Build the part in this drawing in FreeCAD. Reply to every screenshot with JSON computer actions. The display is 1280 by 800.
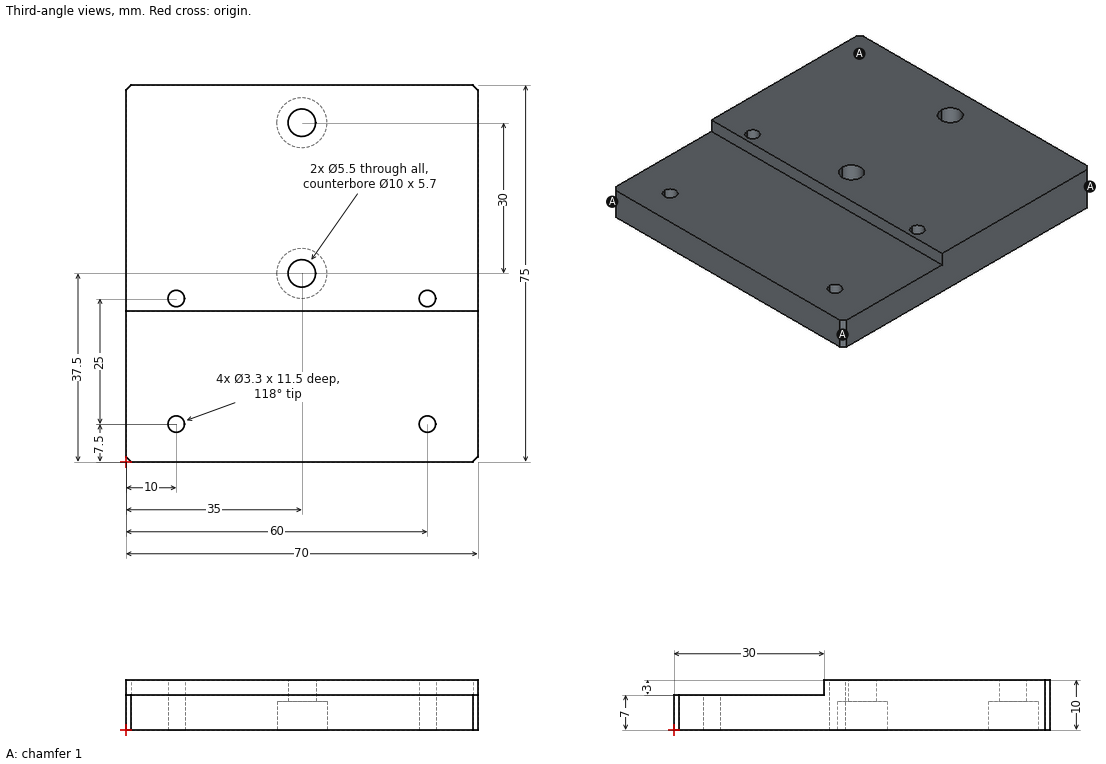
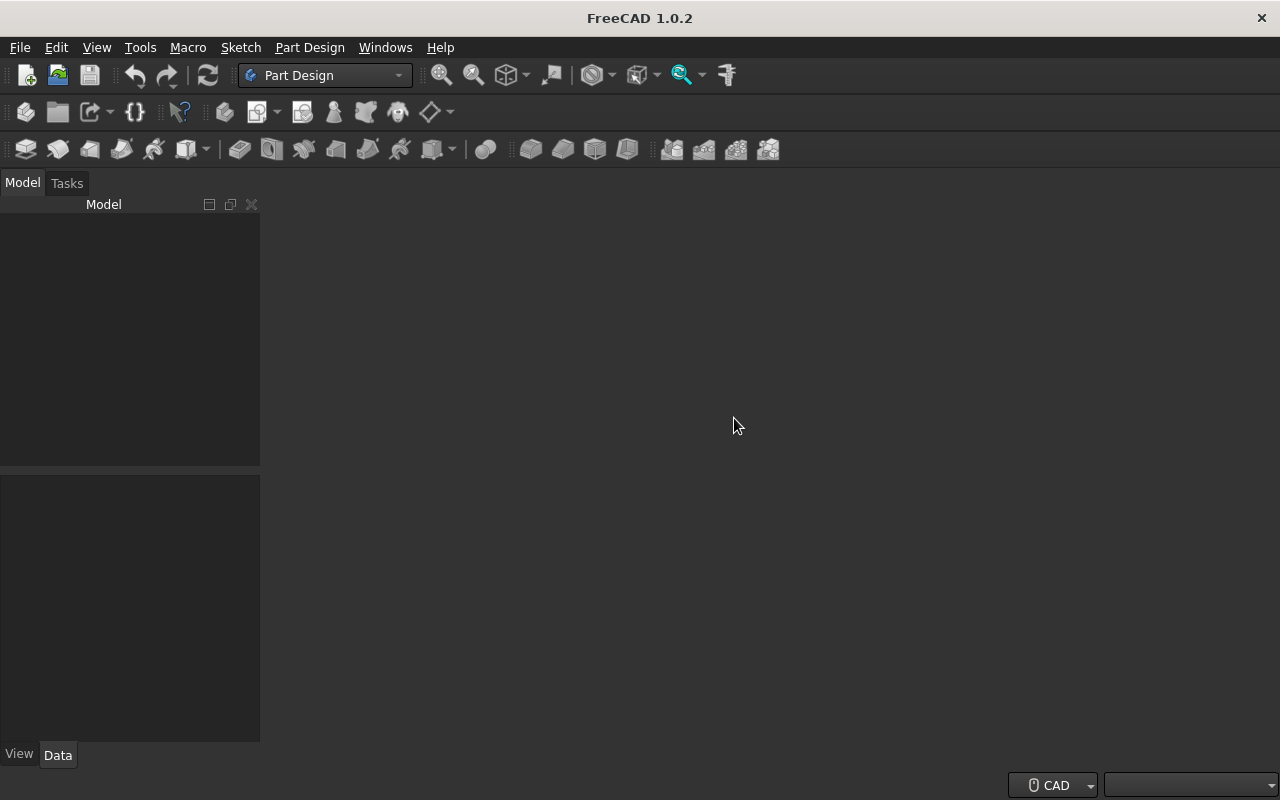
{"action": "left_click", "coordinate": [26, 76]}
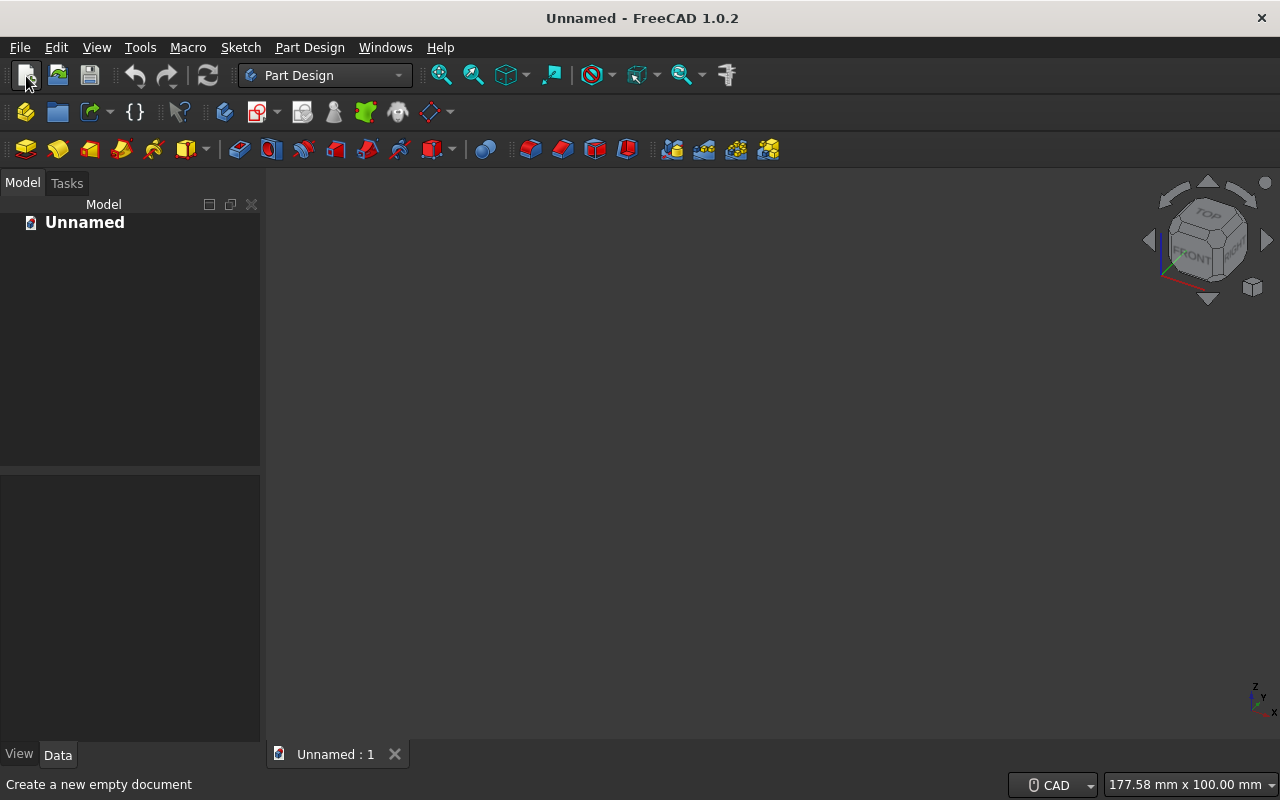
{"action": "left_click", "coordinate": [258, 112]}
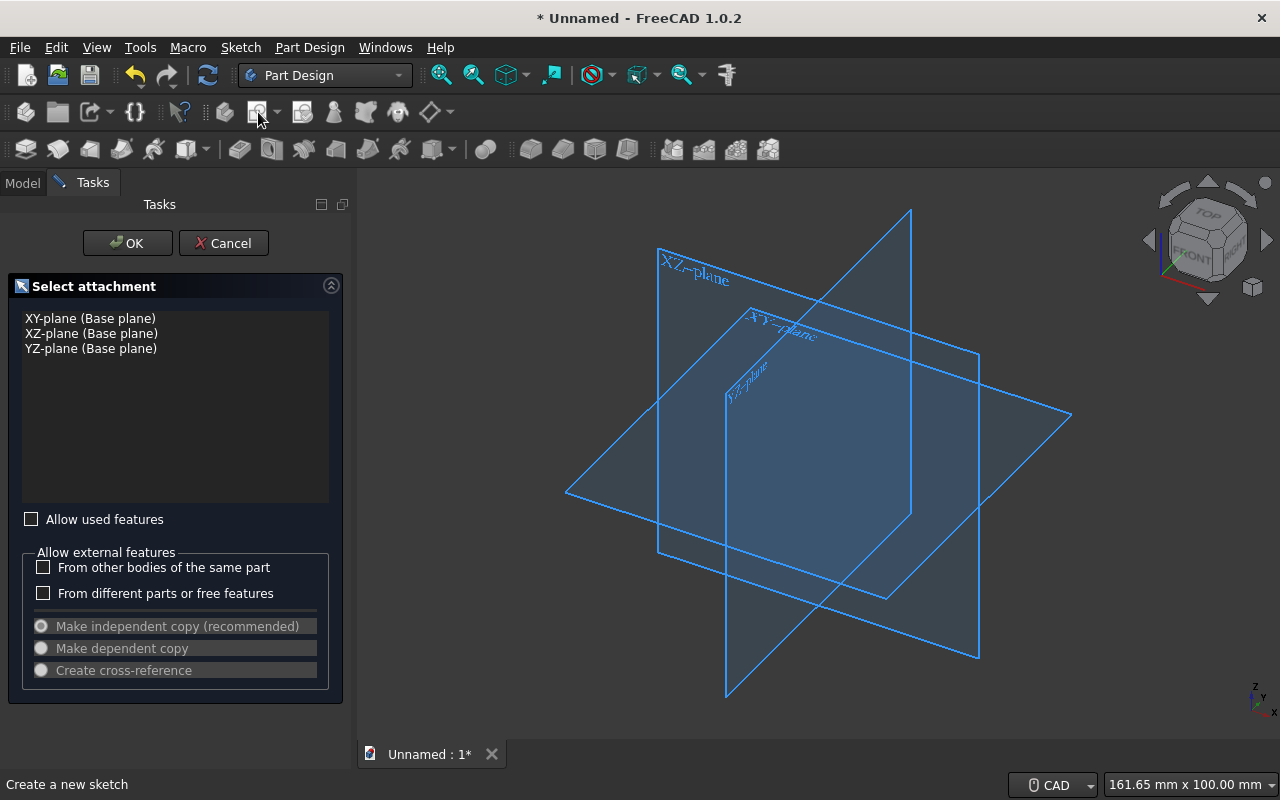
{"action": "left_click", "coordinate": [82, 318]}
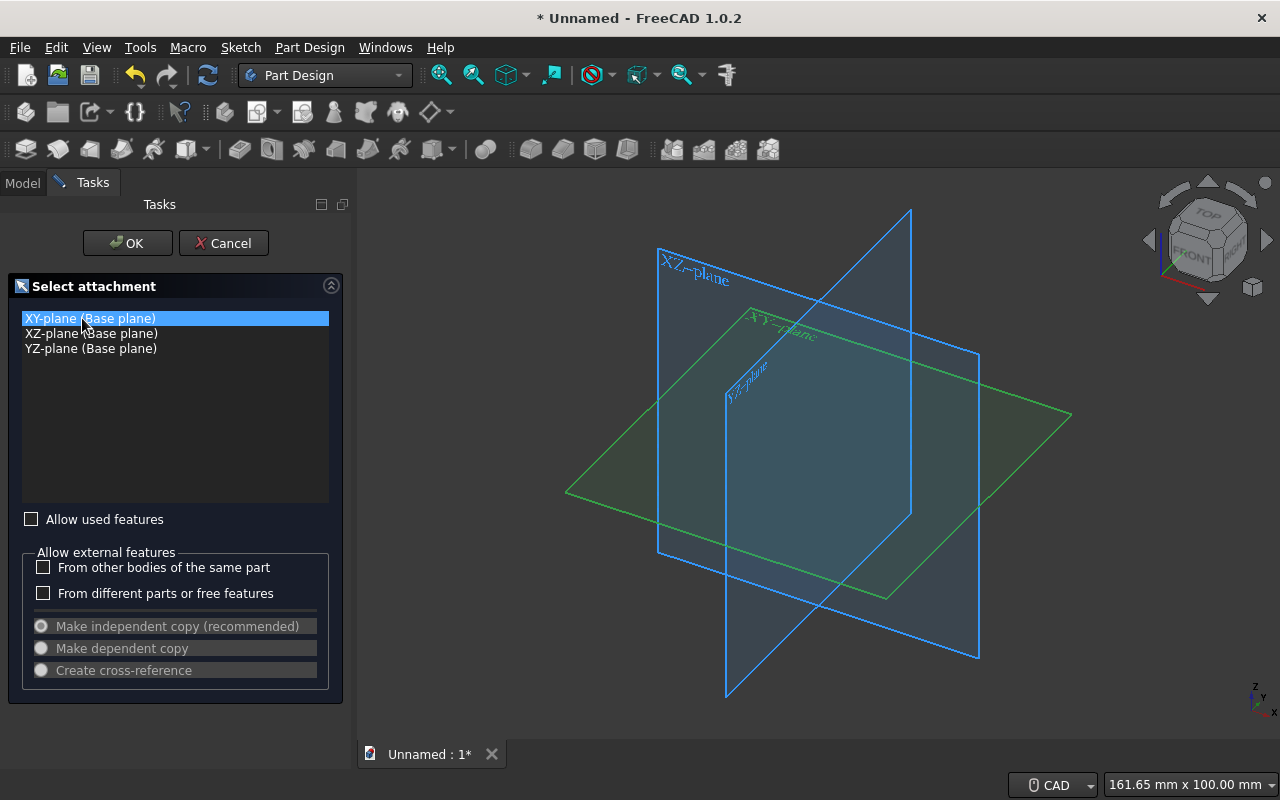
{"action": "left_click", "coordinate": [128, 243]}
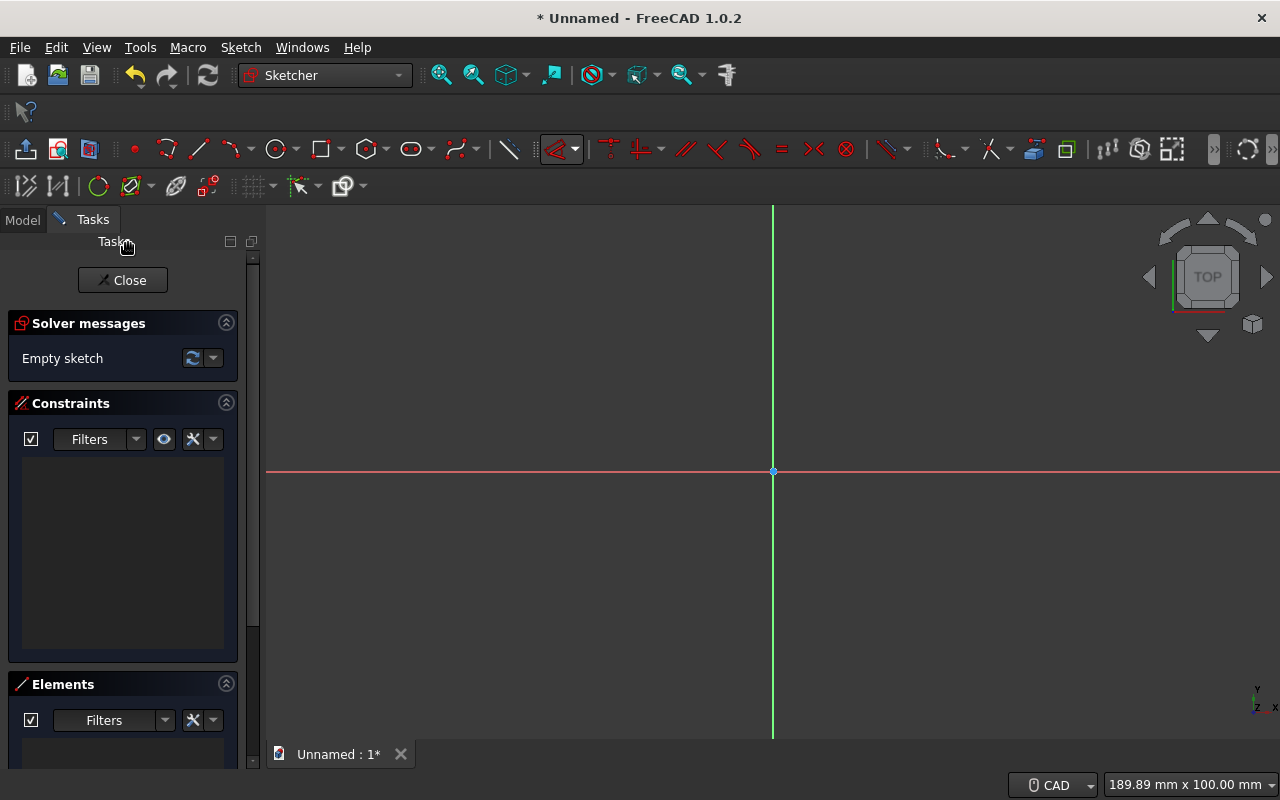
{"action": "scroll", "coordinate": [294, 711], "scroll_direction": "down", "scroll_amount": 2}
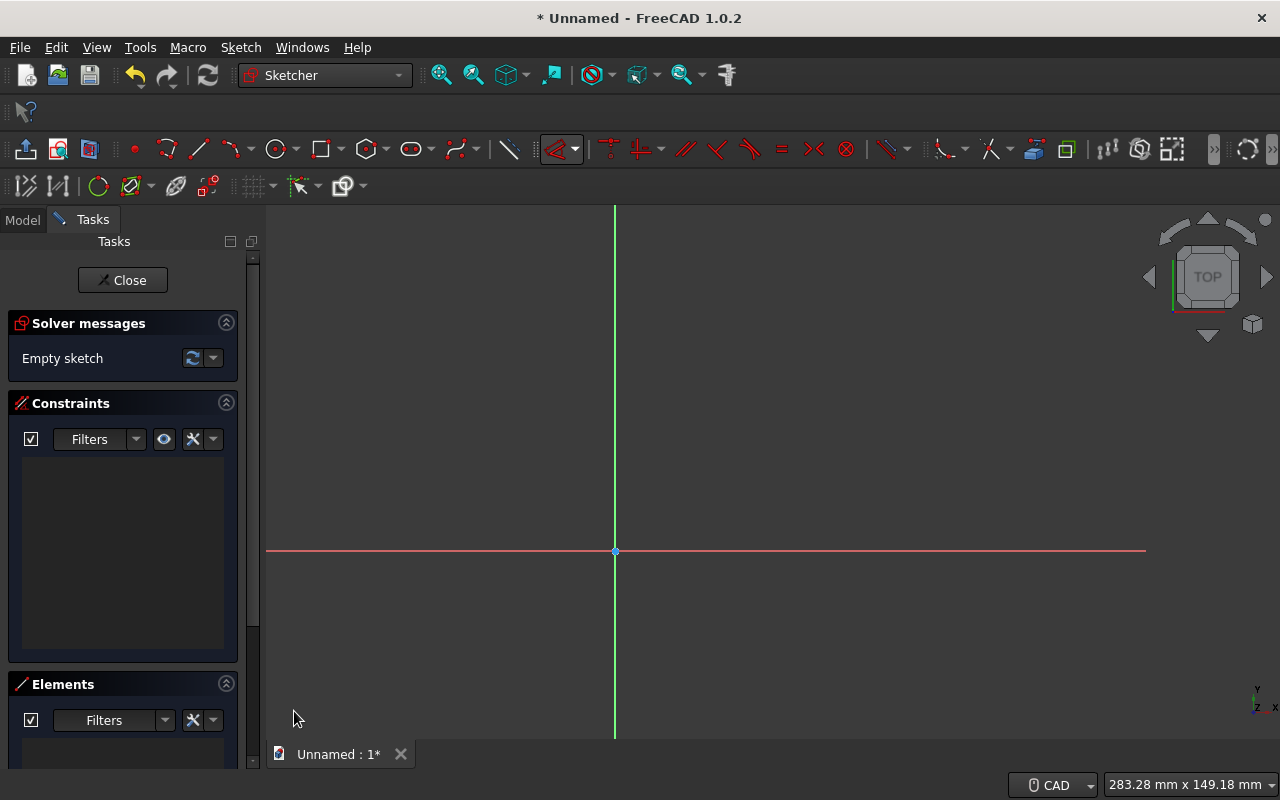
{"action": "key", "text": "g r"}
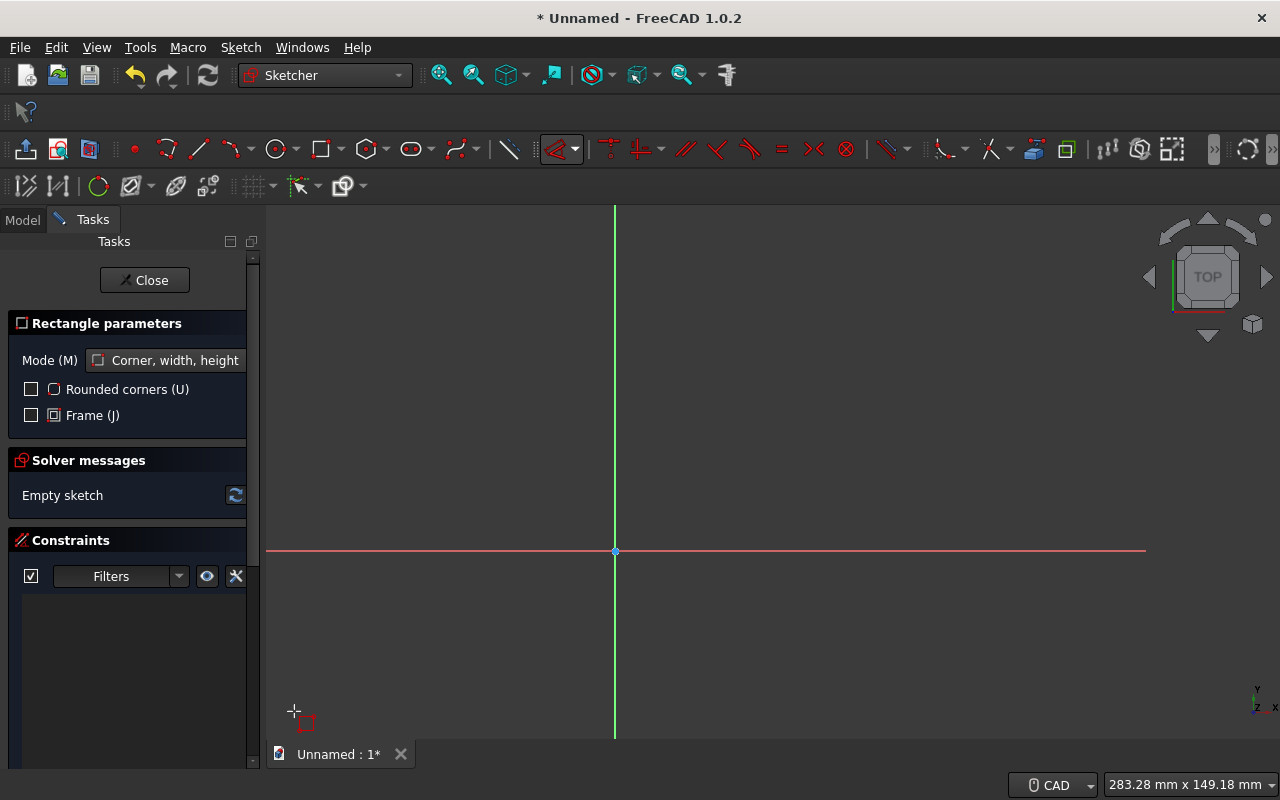
{"action": "left_click", "coordinate": [615, 551]}
{"action": "mouse_move", "coordinate": [866, 283]}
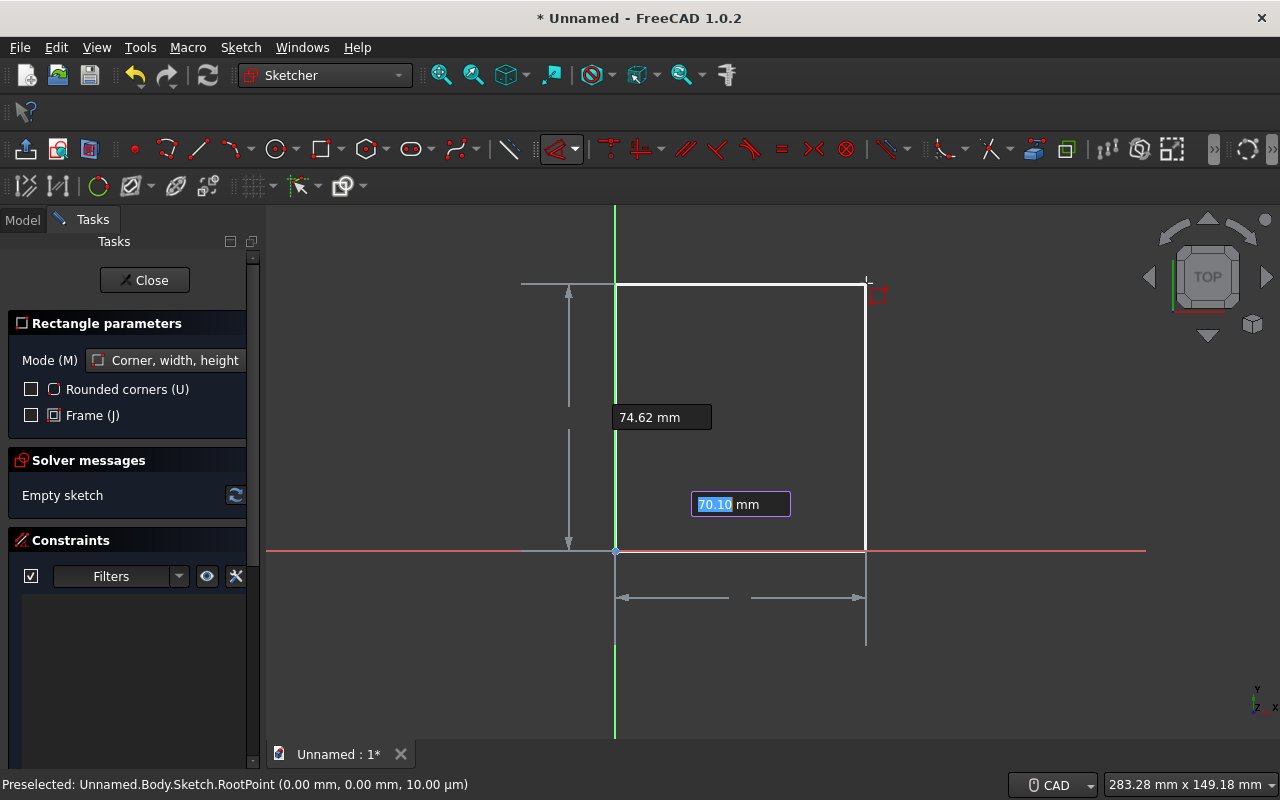
{"action": "type", "text": "70"}
{"action": "key", "text": "Tab"}
{"action": "type", "text": "75"}
{"action": "key", "text": "Return"}
{"action": "key", "text": "Escape"}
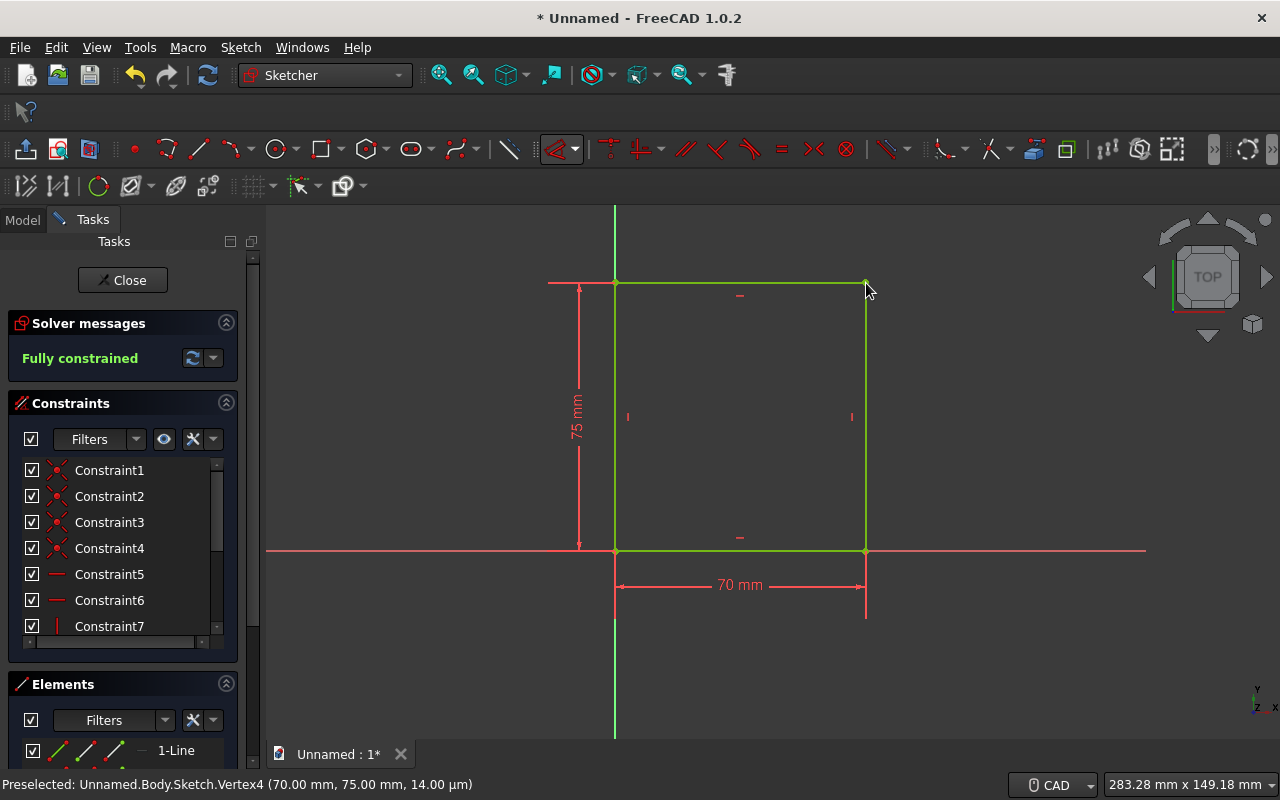
{"action": "left_click", "coordinate": [123, 280]}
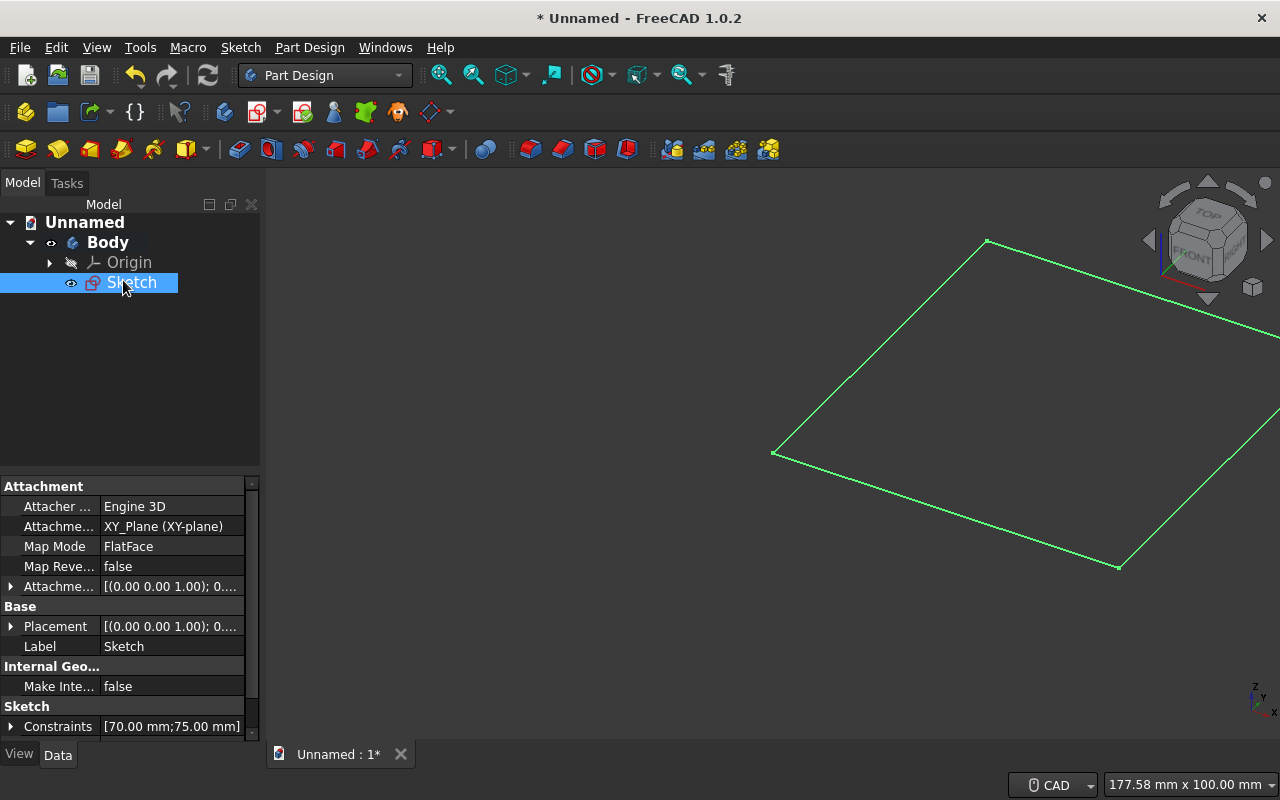
{"action": "left_click", "coordinate": [26, 150]}